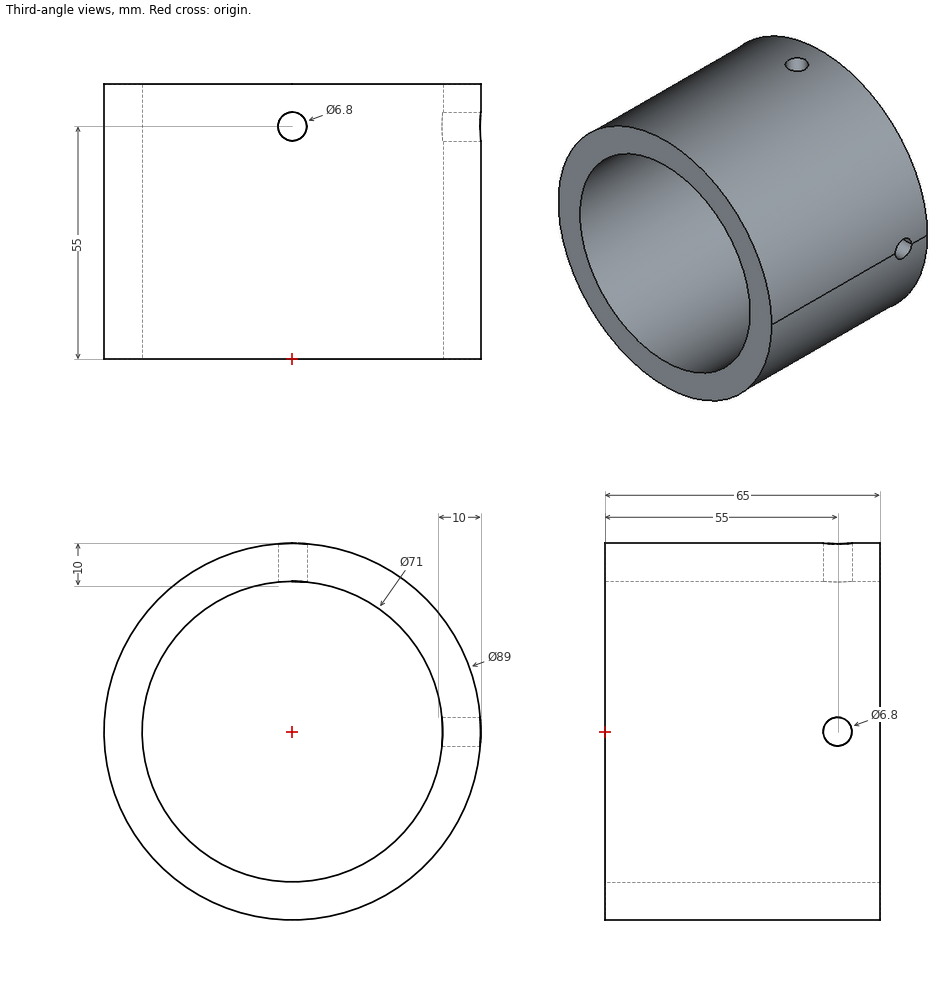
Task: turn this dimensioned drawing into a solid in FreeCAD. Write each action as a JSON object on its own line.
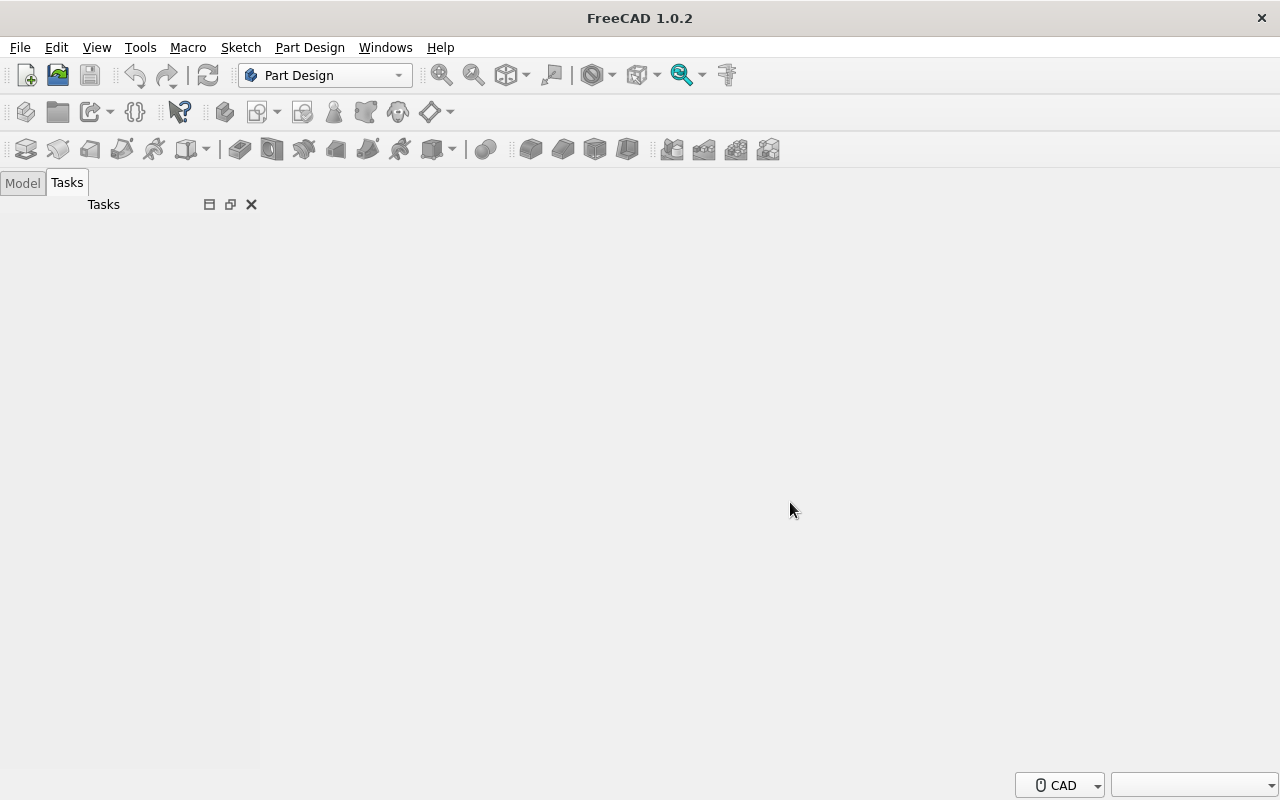
{"action": "key", "text": "ctrl+n"}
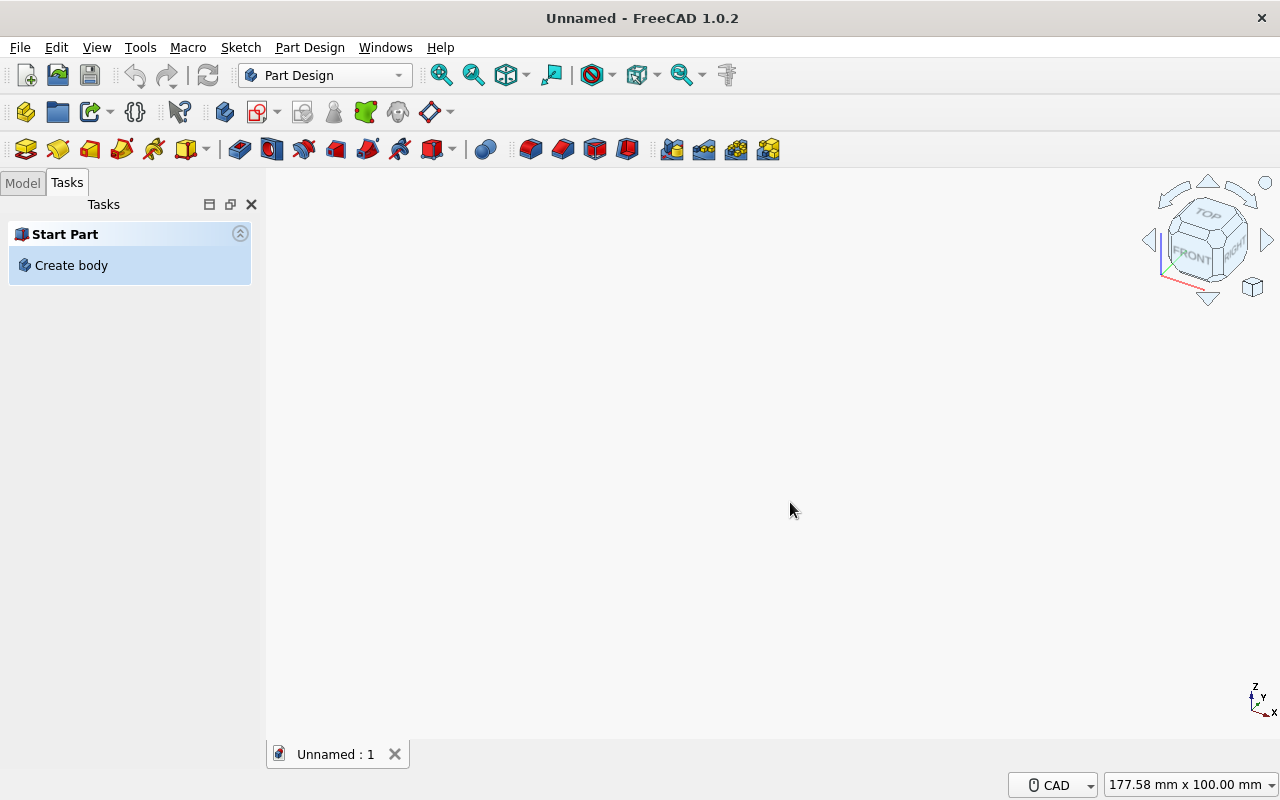
{"action": "left_click", "coordinate": [258, 112]}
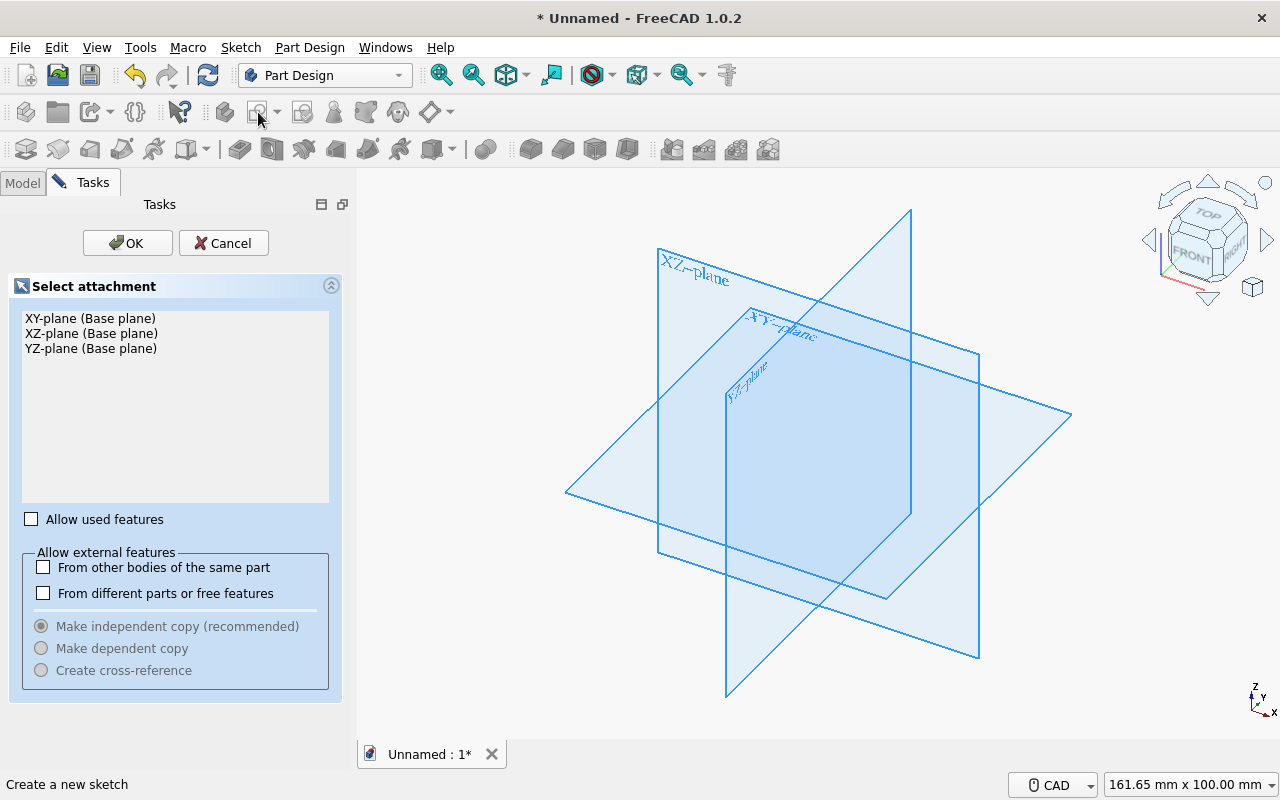
{"action": "left_click", "coordinate": [82, 334]}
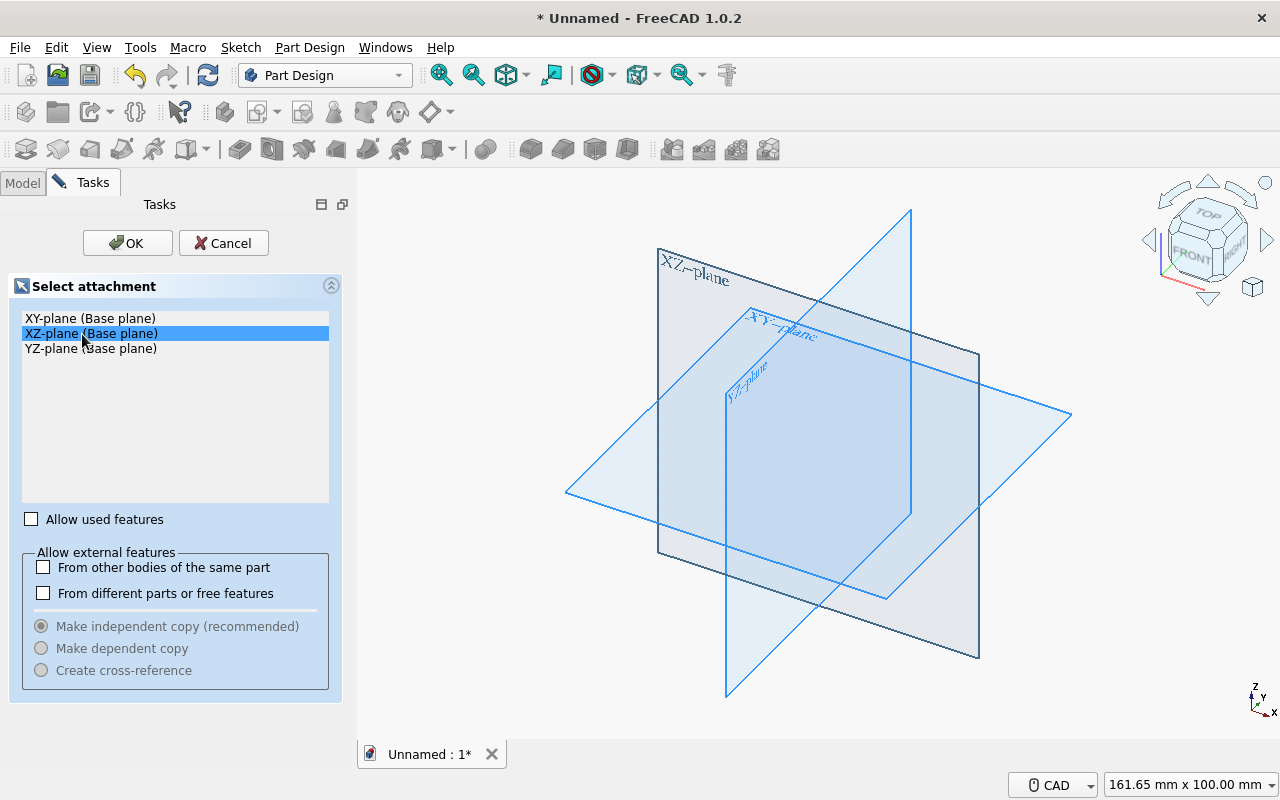
{"action": "left_click", "coordinate": [128, 243]}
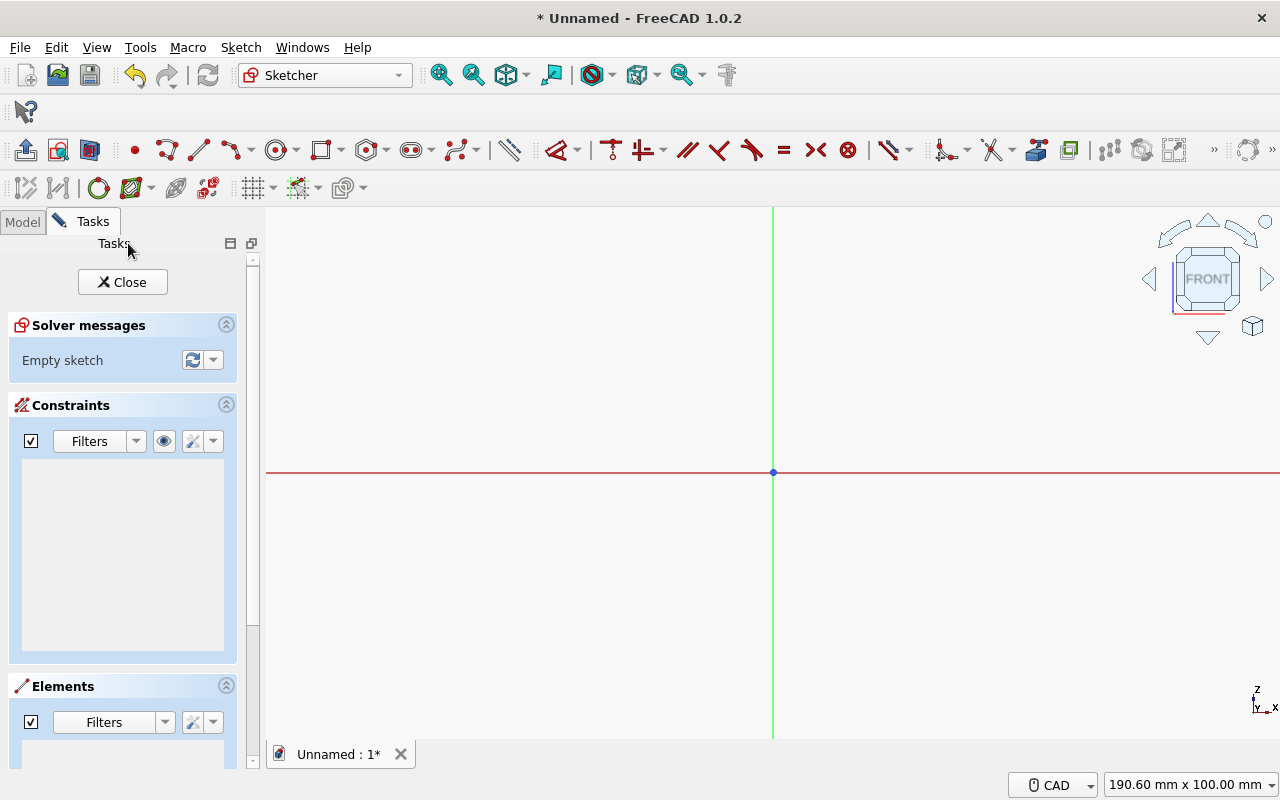
{"action": "scroll", "coordinate": [565, 473], "scroll_direction": "down", "scroll_amount": 2}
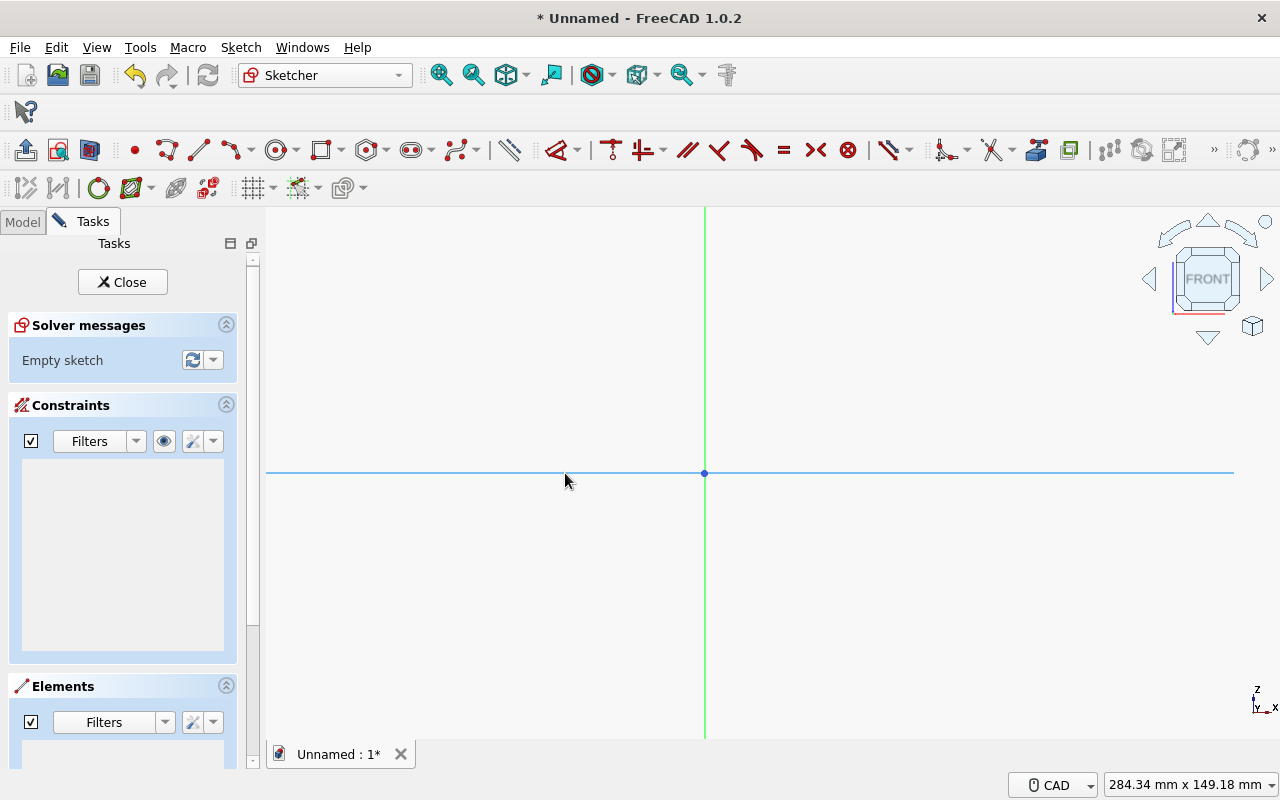
{"action": "key", "text": "g c"}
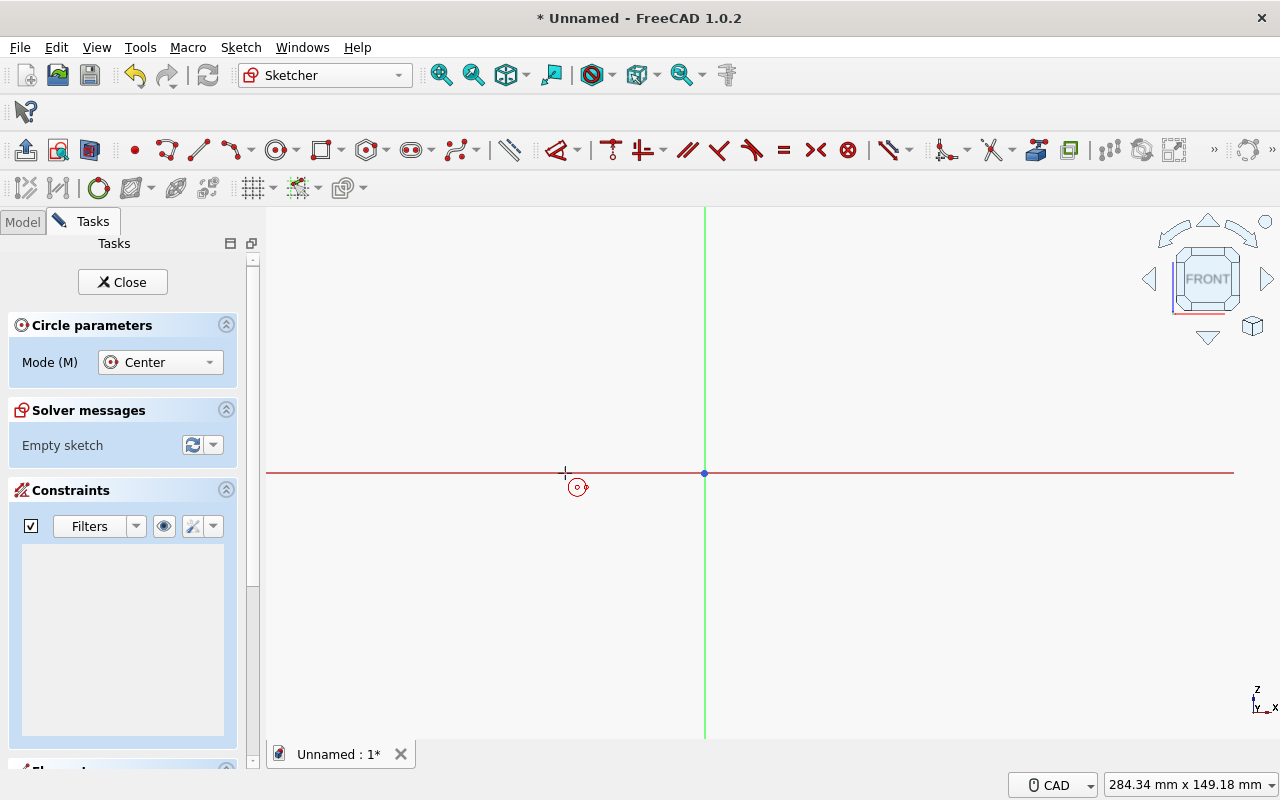
{"action": "left_click", "coordinate": [705, 473]}
{"action": "mouse_move", "coordinate": [817, 361]}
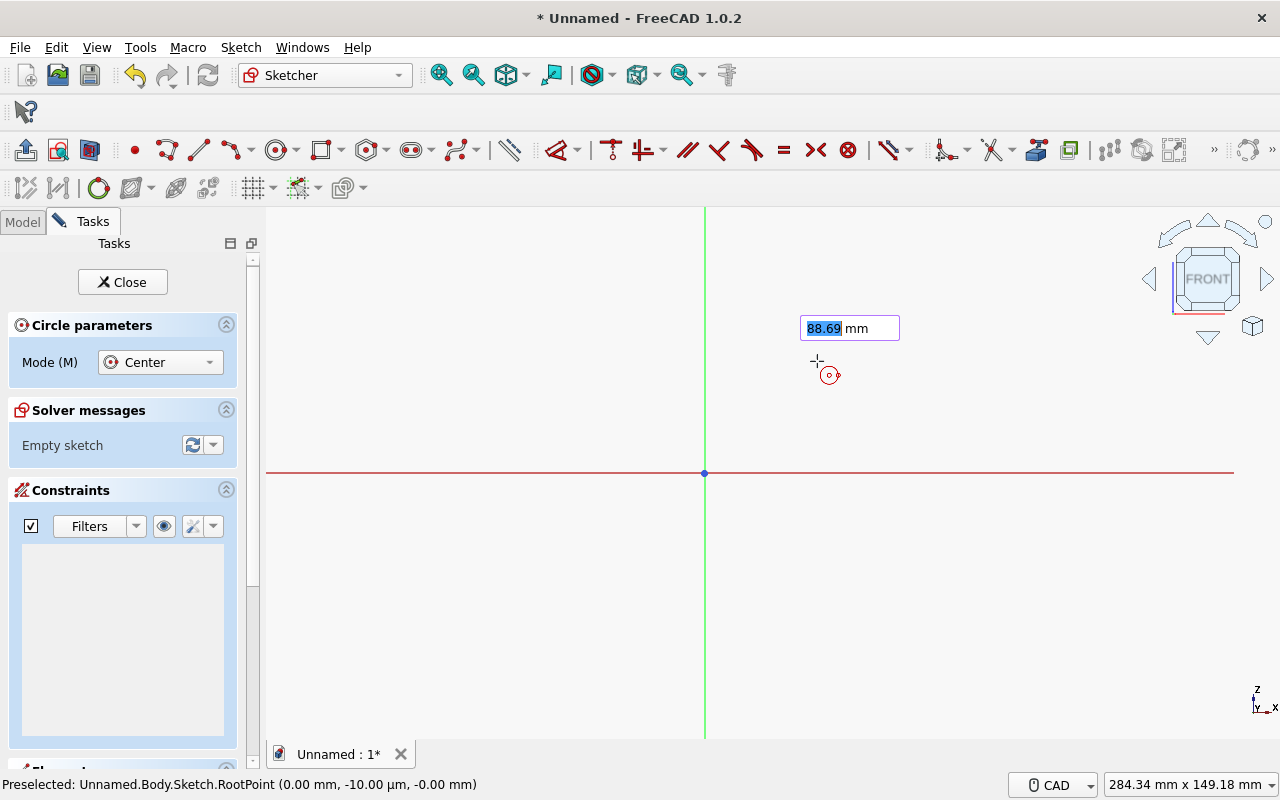
{"action": "type", "text": "89"}
{"action": "key", "text": "Return"}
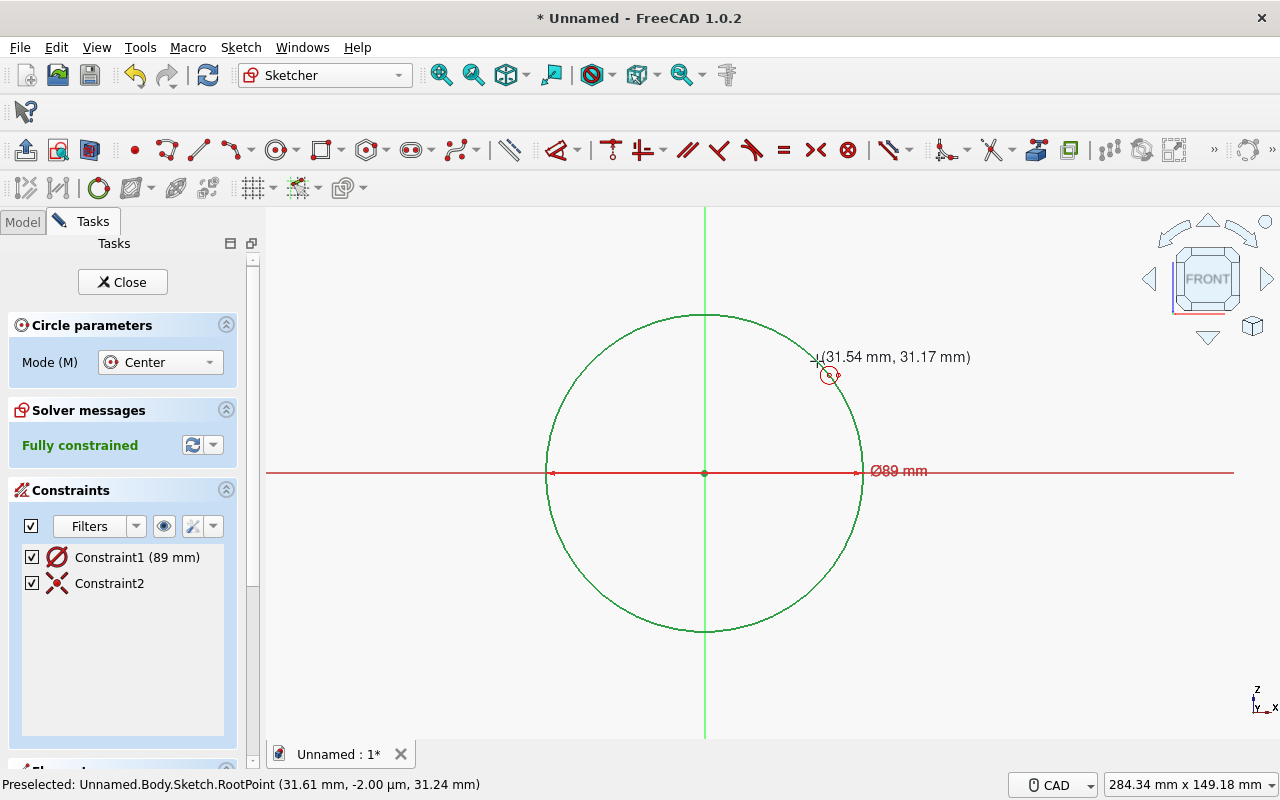
{"action": "left_click", "coordinate": [705, 473]}
{"action": "mouse_move", "coordinate": [794, 384]}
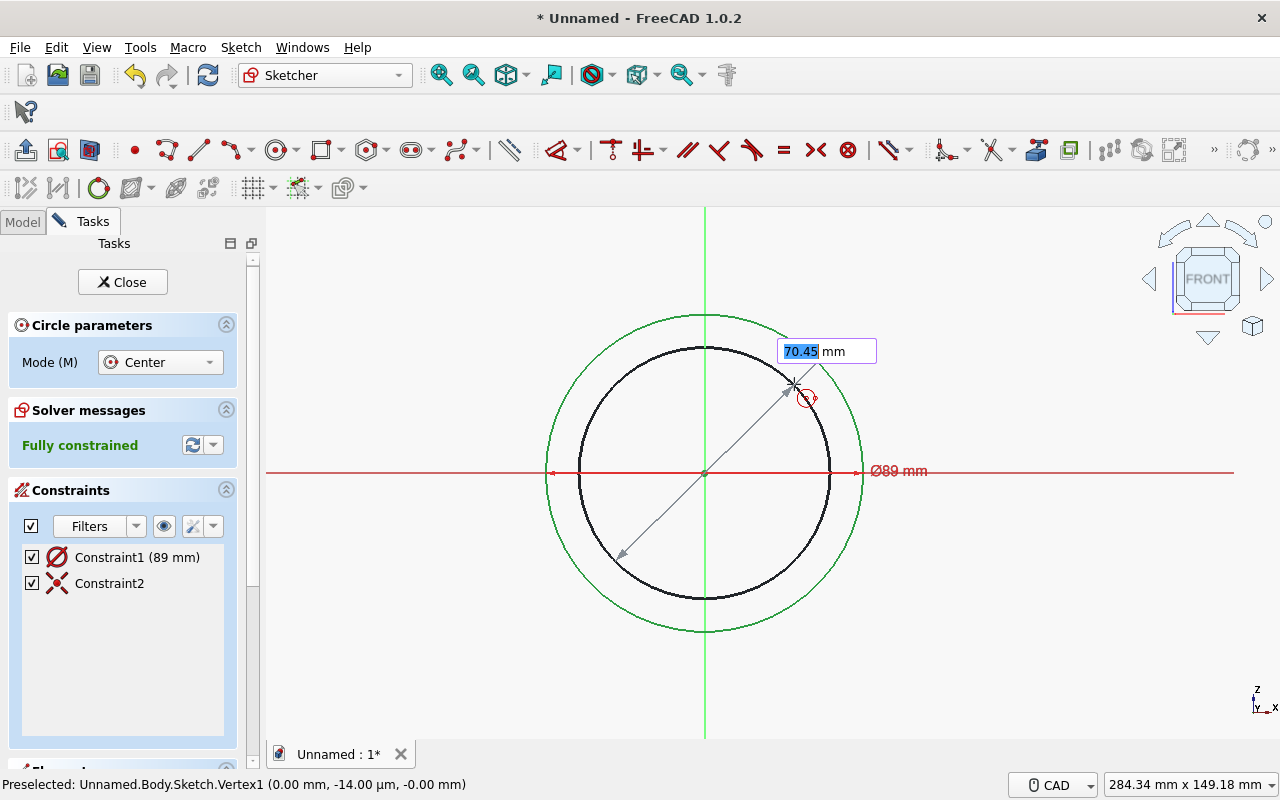
{"action": "type", "text": "71"}
{"action": "key", "text": "Return"}
{"action": "key", "text": "Escape"}